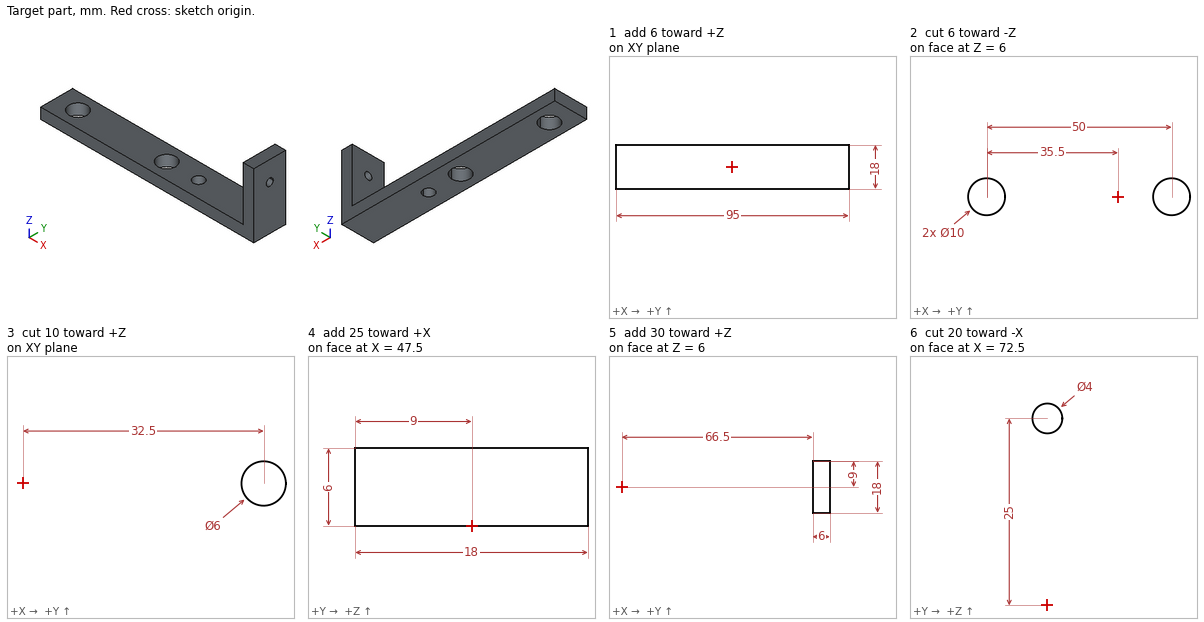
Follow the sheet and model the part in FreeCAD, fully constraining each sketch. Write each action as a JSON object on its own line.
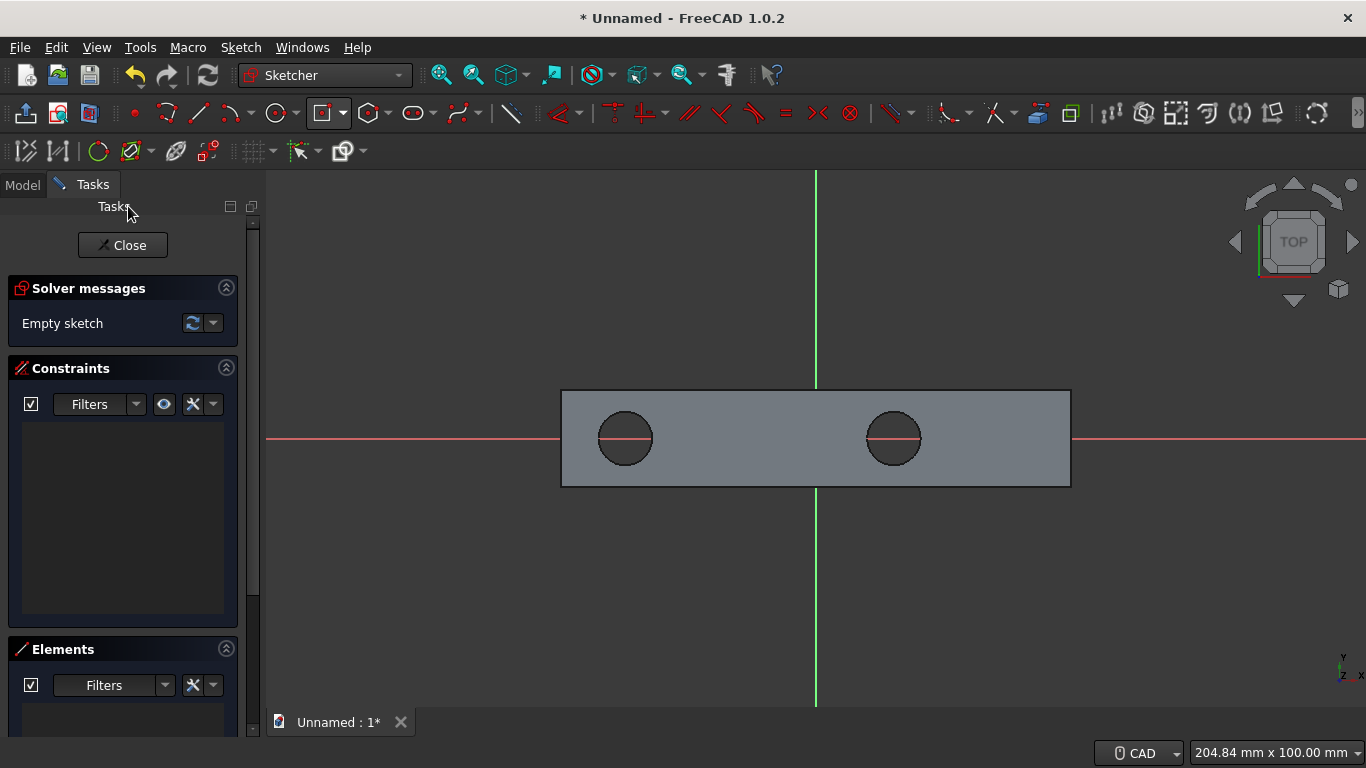
{"action": "key", "text": "q s"}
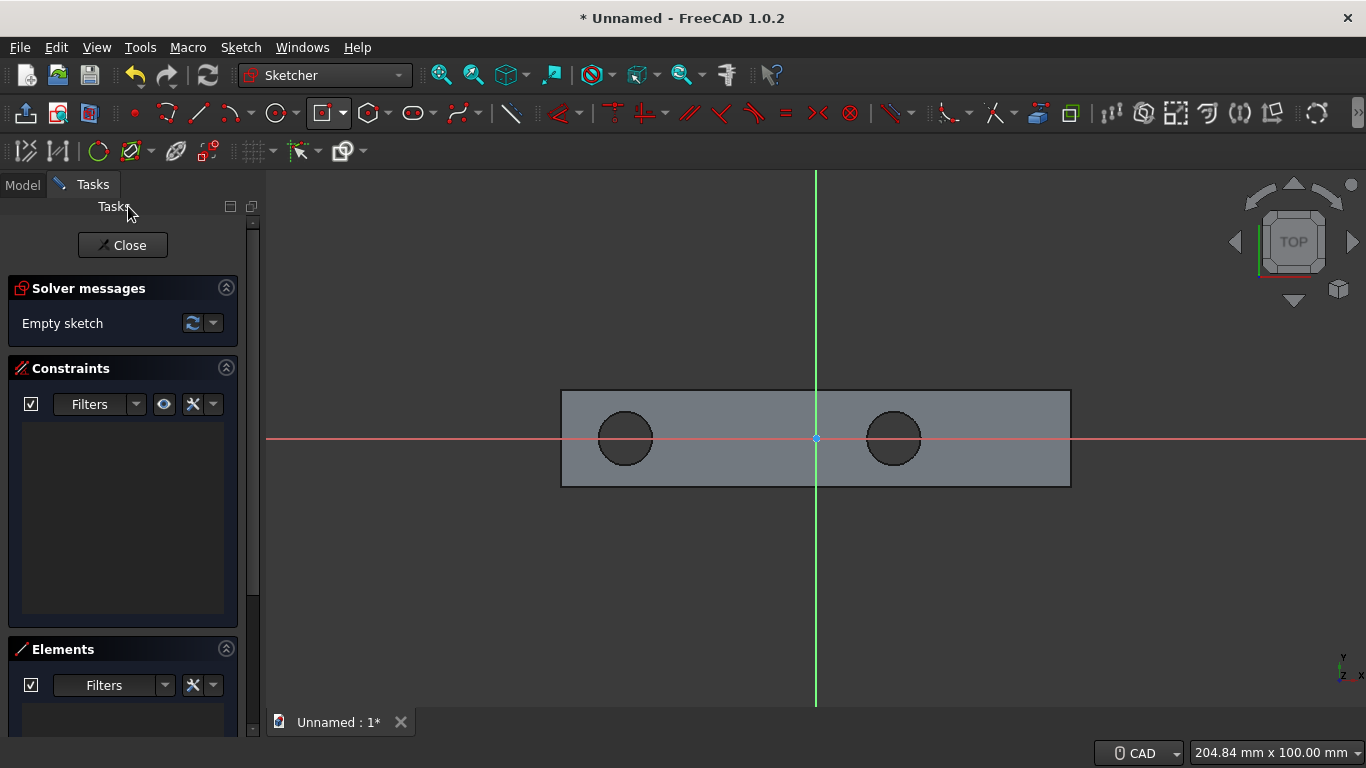
{"action": "scroll", "coordinate": [1015, 438], "scroll_direction": "up", "scroll_amount": 12}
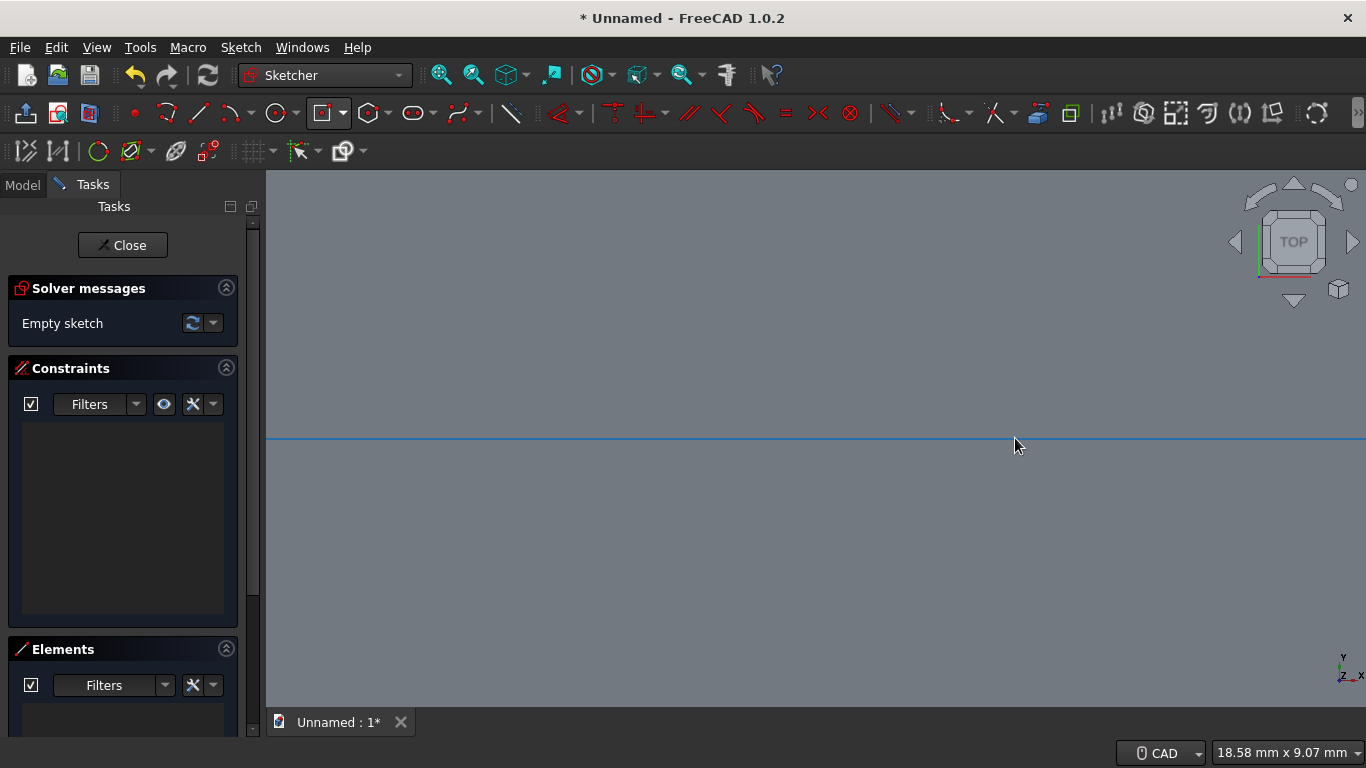
{"action": "key", "text": "g c"}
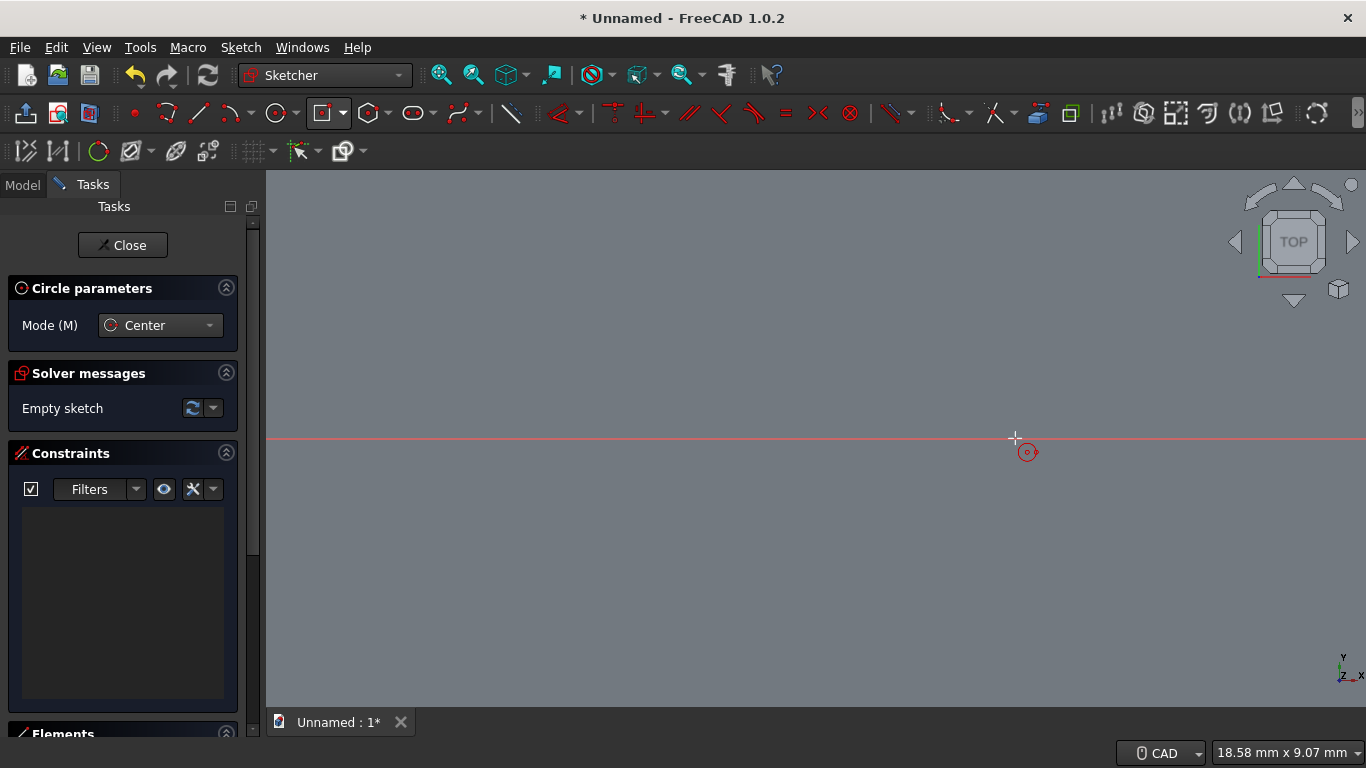
{"action": "left_click", "coordinate": [738, 438]}
{"action": "left_click", "coordinate": [864, 313]}
{"action": "key", "text": "Escape"}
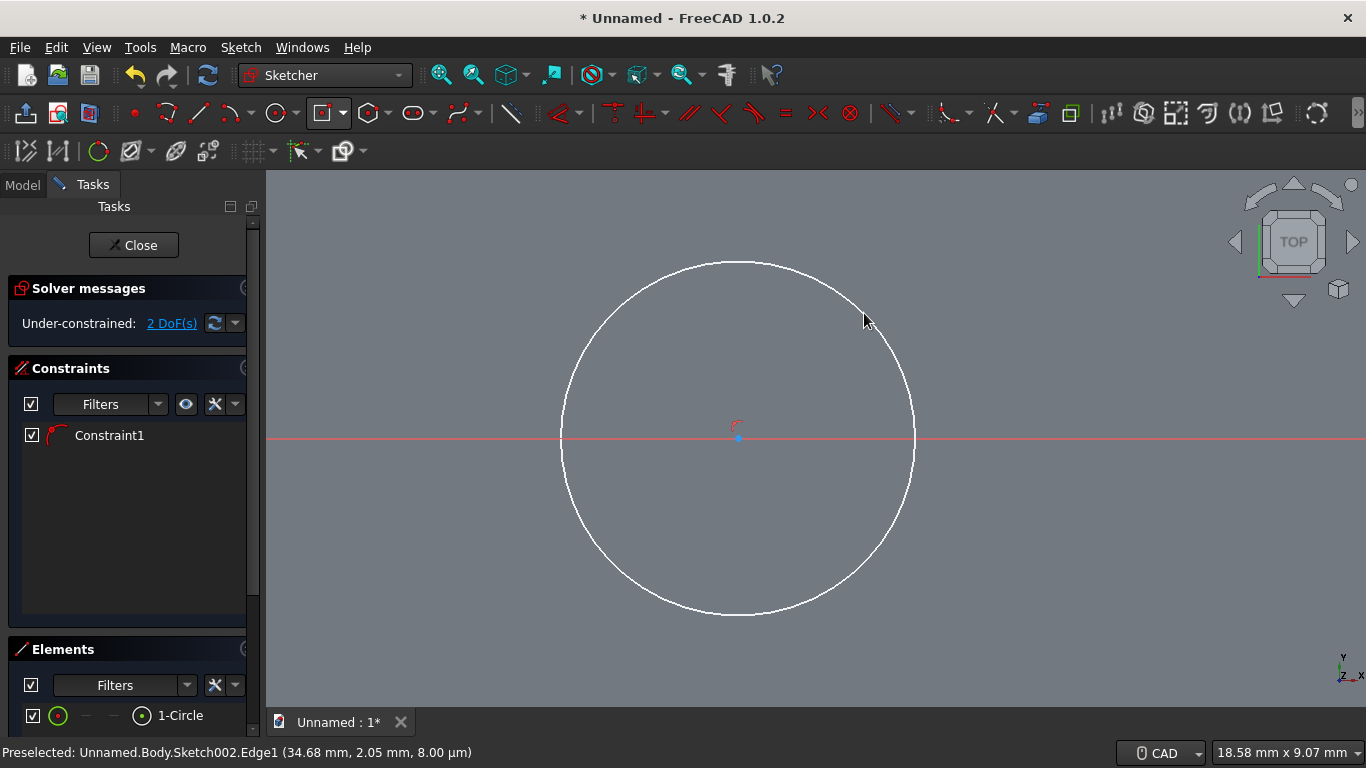
{"action": "left_click", "coordinate": [558, 114]}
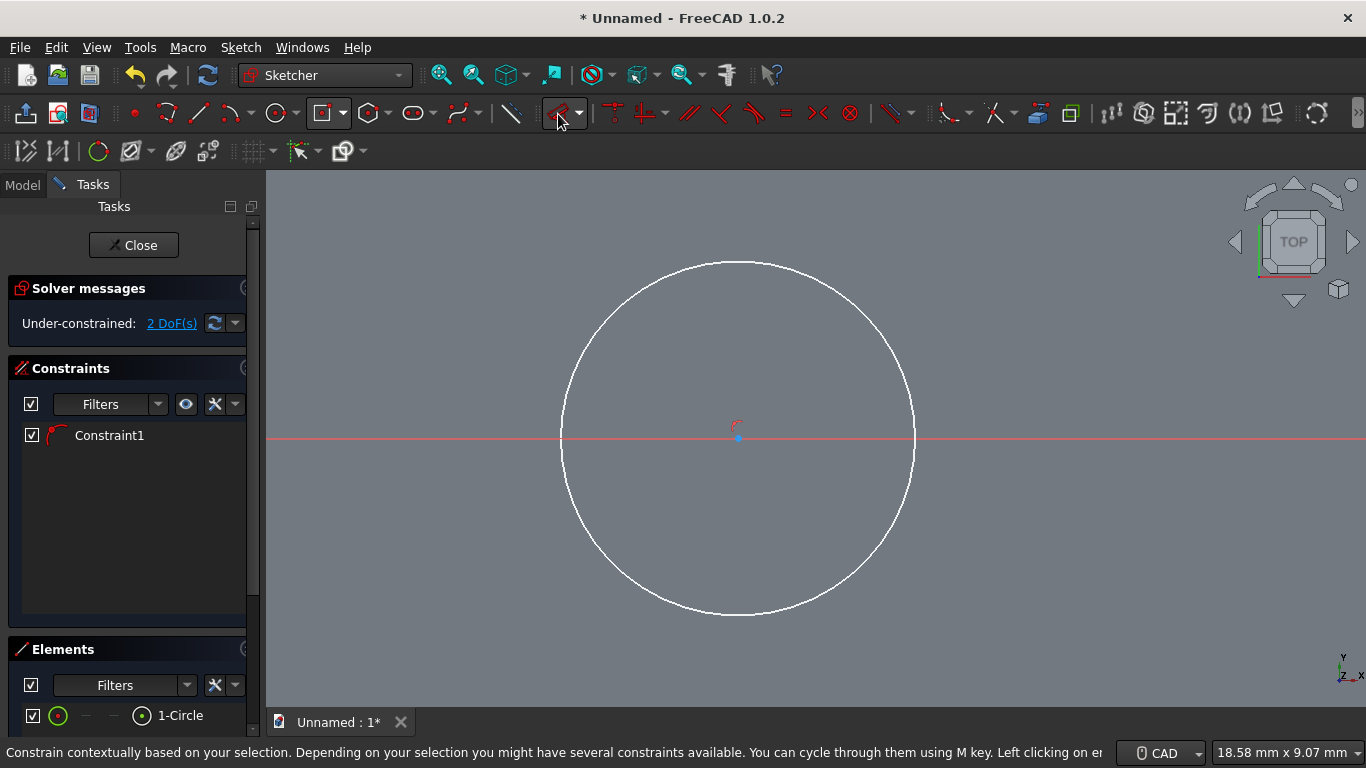
{"action": "left_click", "coordinate": [863, 313]}
{"action": "left_click", "coordinate": [886, 290]}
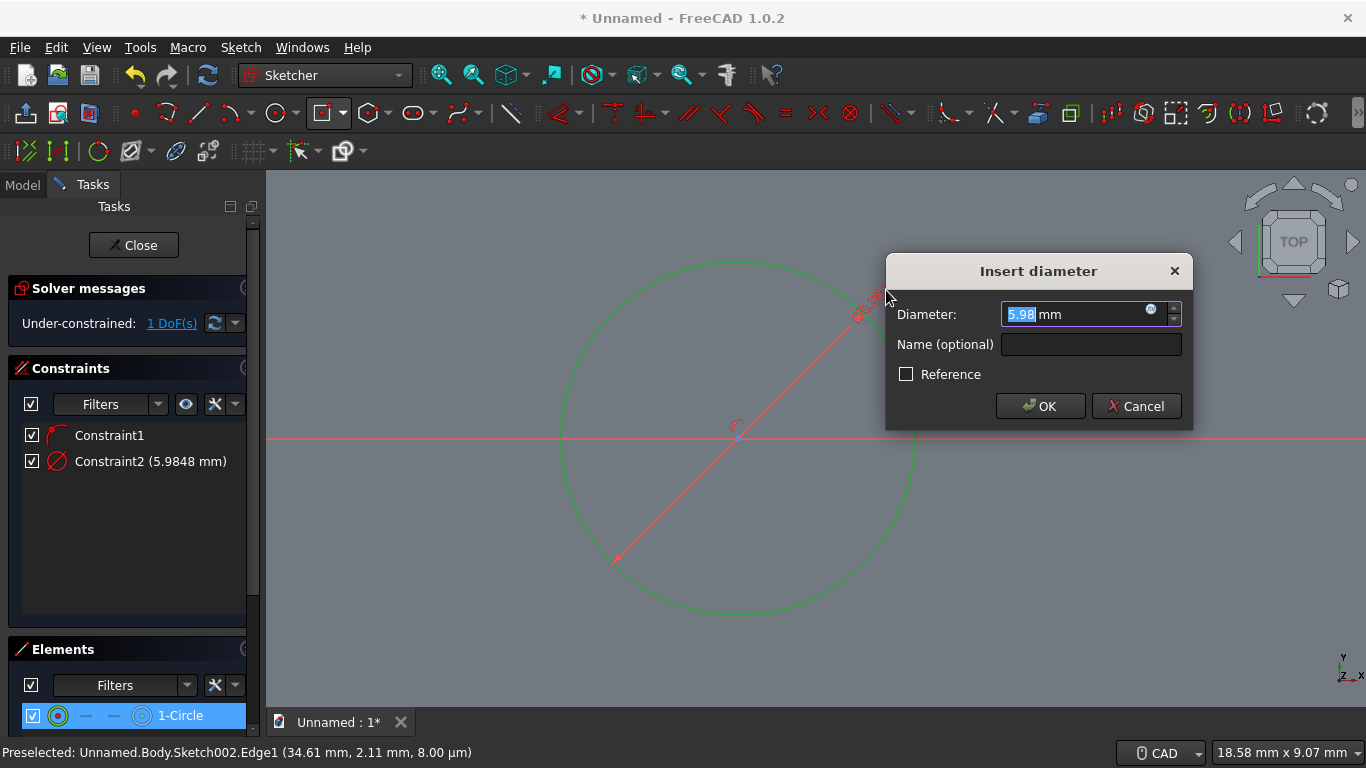
{"action": "type", "text": "6"}
{"action": "key", "text": "Return"}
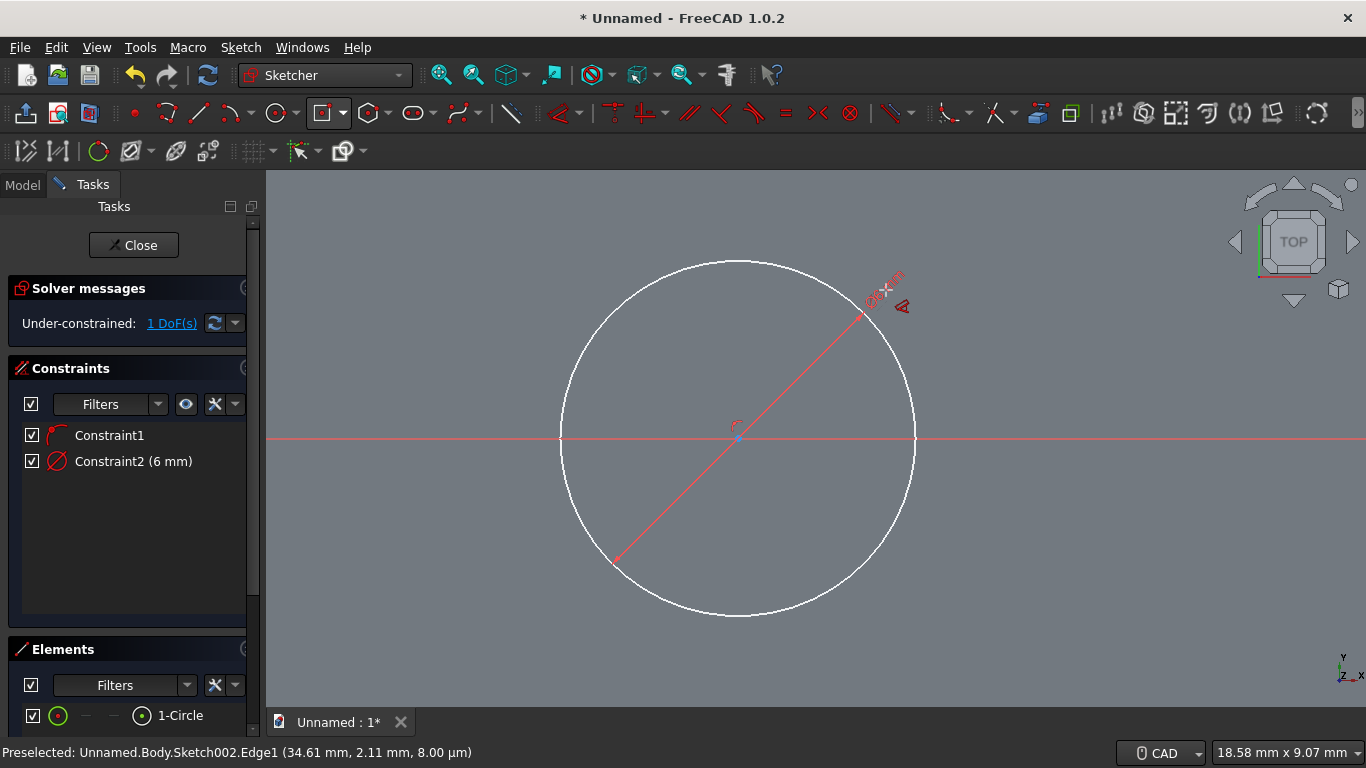
{"action": "left_click", "coordinate": [738, 438]}
{"action": "left_click", "coordinate": [516, 472]}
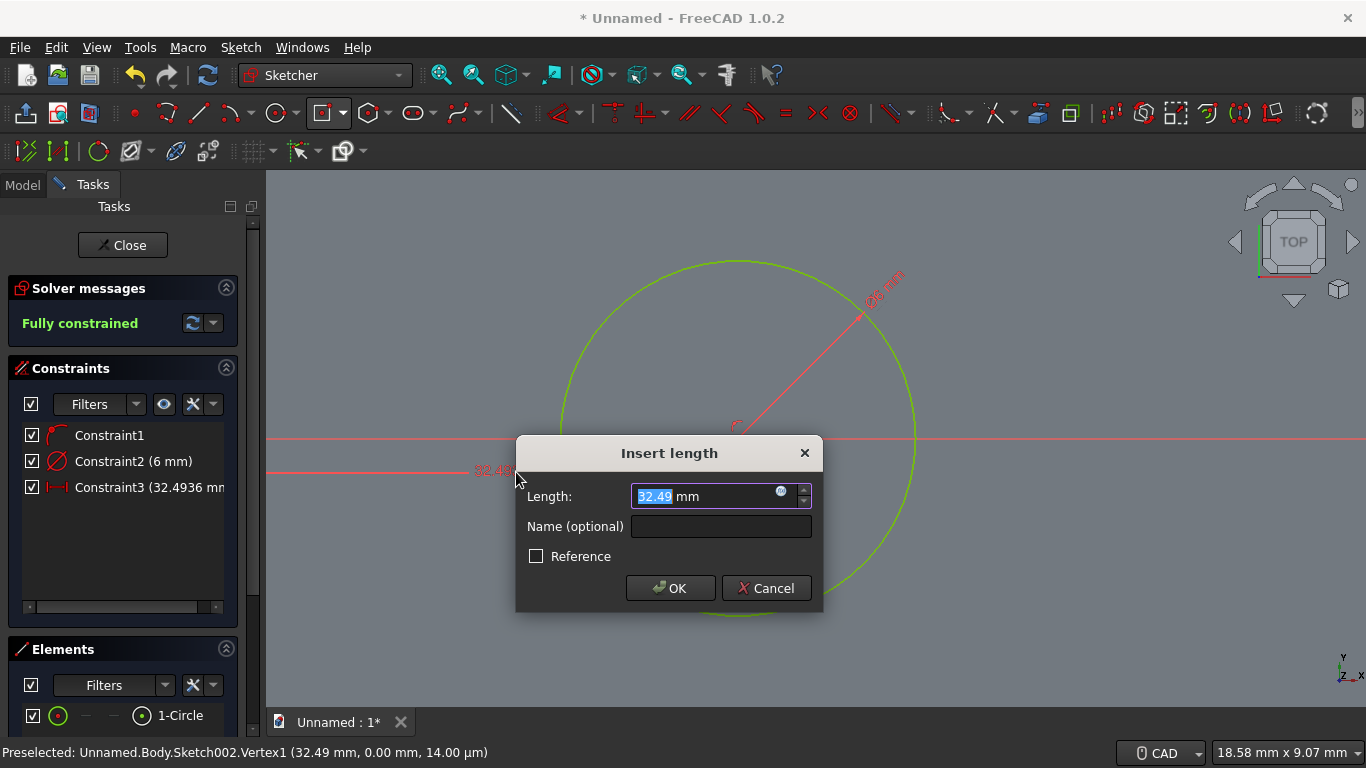
{"action": "type", "text": "32.5"}
{"action": "key", "text": "Return"}
{"action": "key", "text": "Escape"}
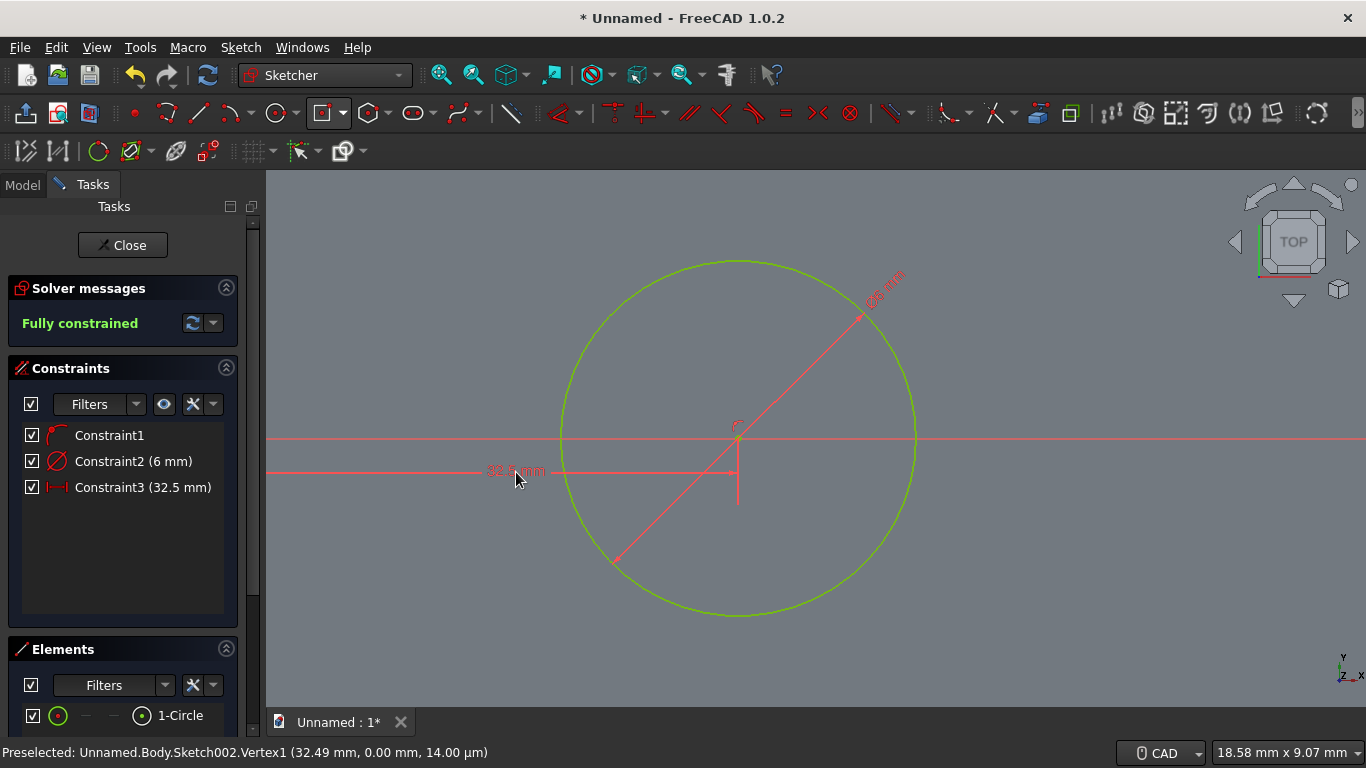
{"action": "left_click", "coordinate": [123, 245]}